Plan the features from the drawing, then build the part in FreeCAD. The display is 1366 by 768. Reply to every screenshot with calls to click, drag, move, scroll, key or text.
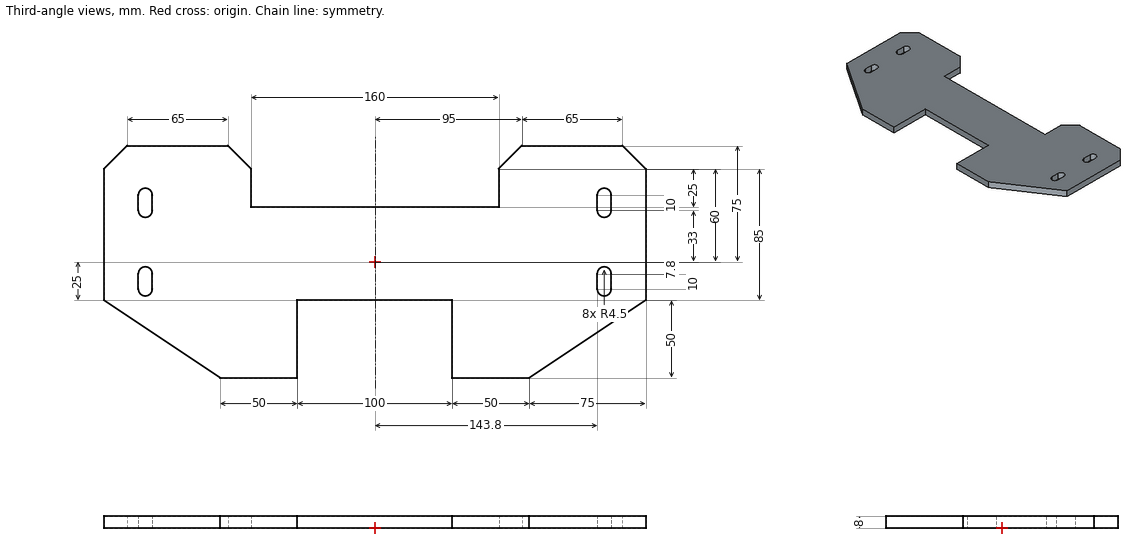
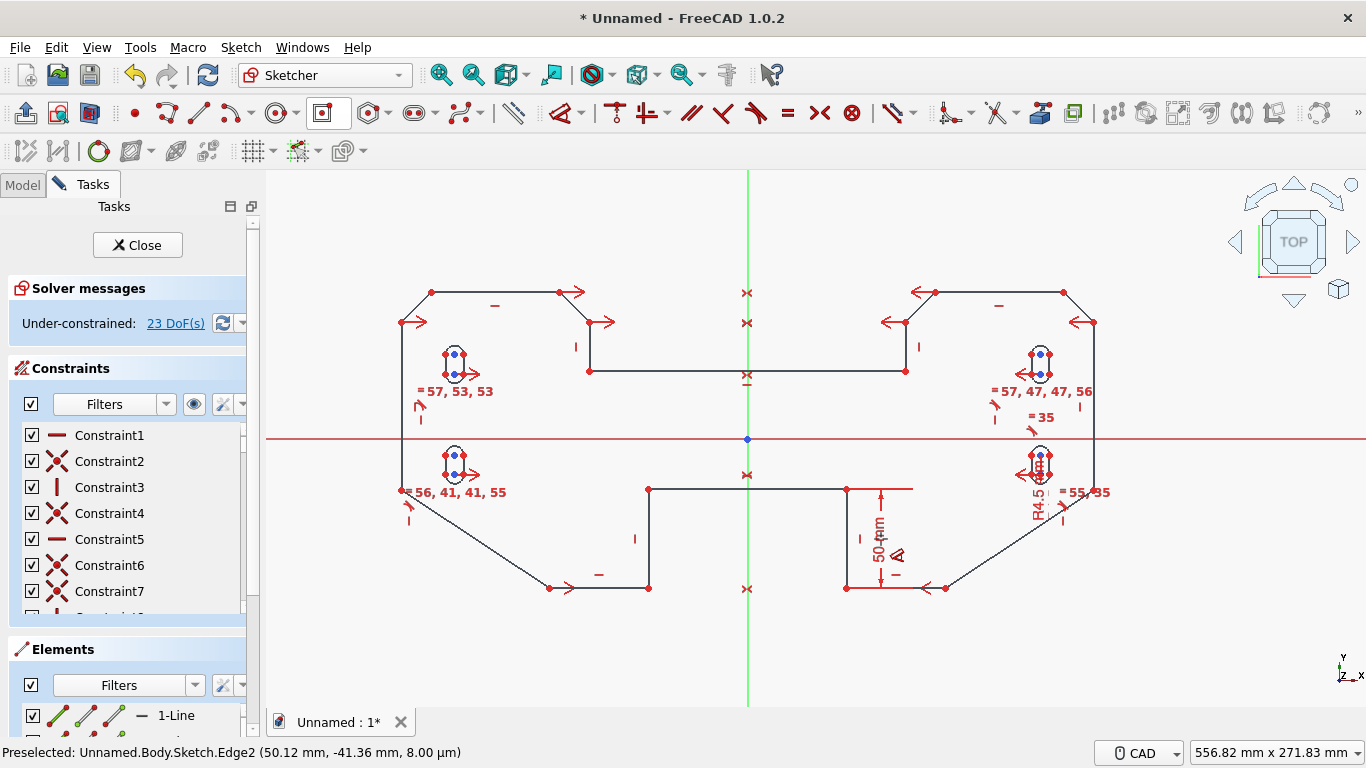
click(876, 588)
click(896, 622)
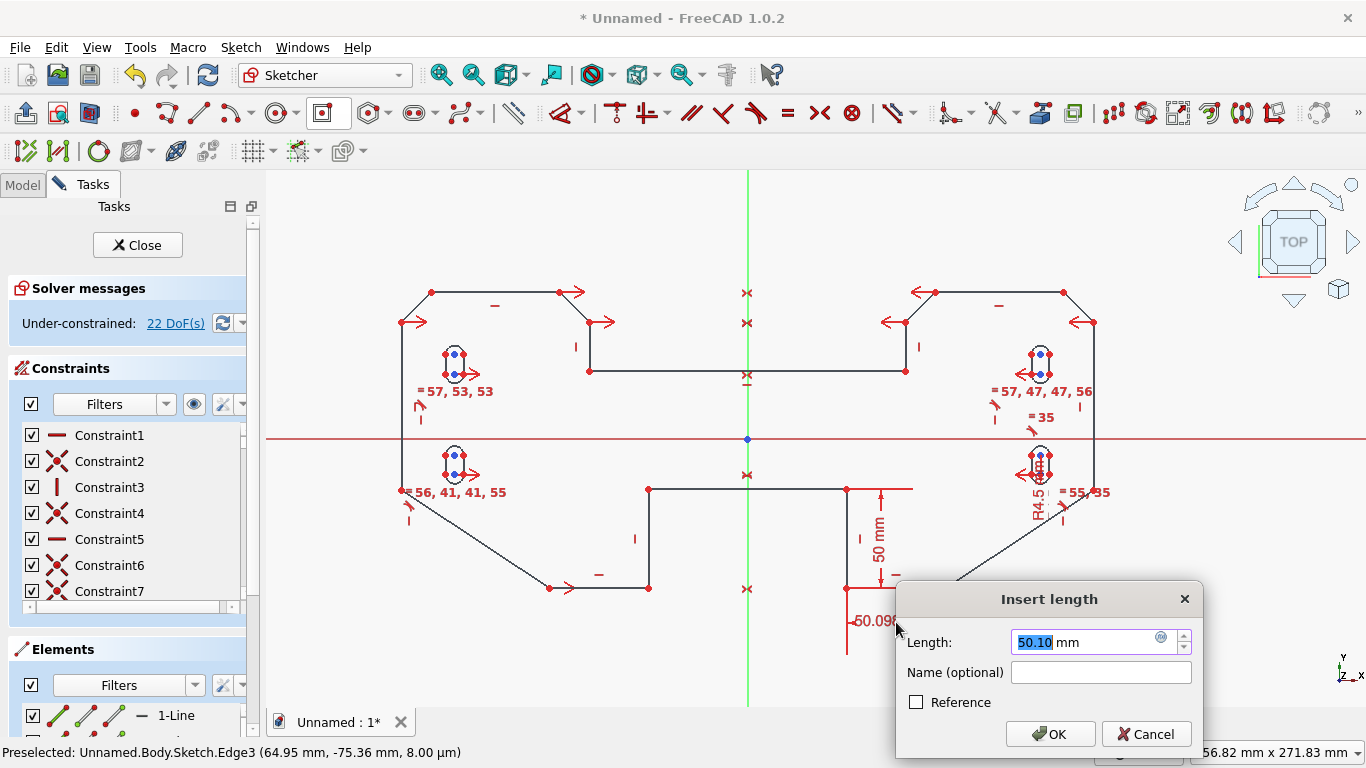
text(50)
key(Return)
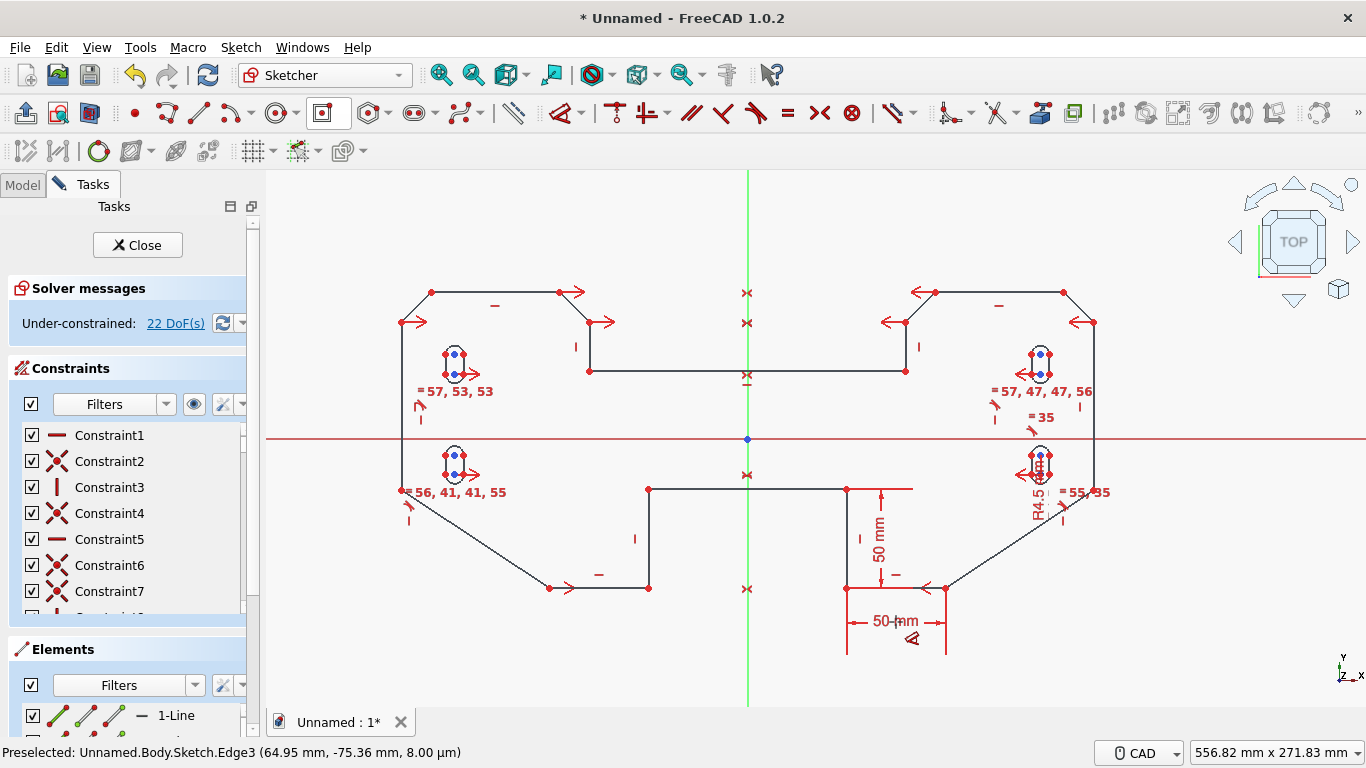
click(1094, 440)
click(1128, 406)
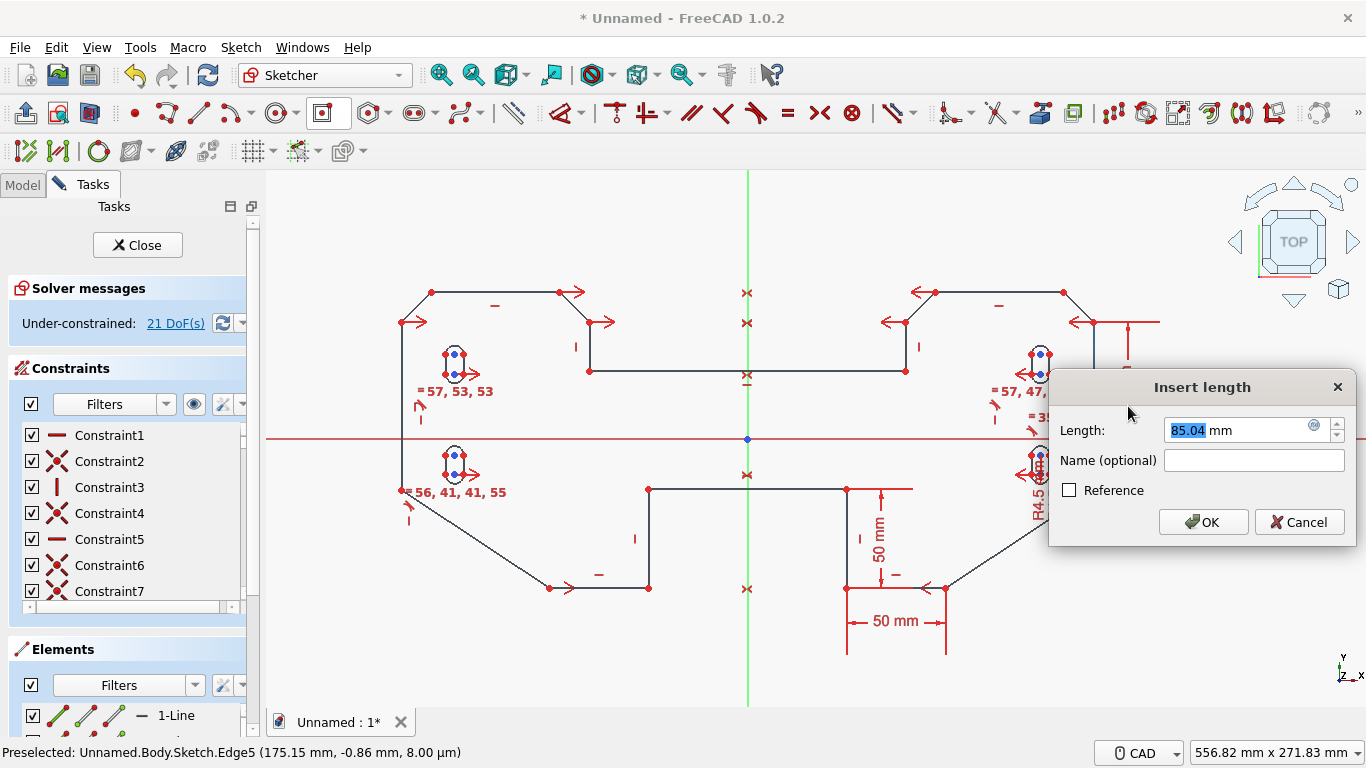
text(85)
key(Return)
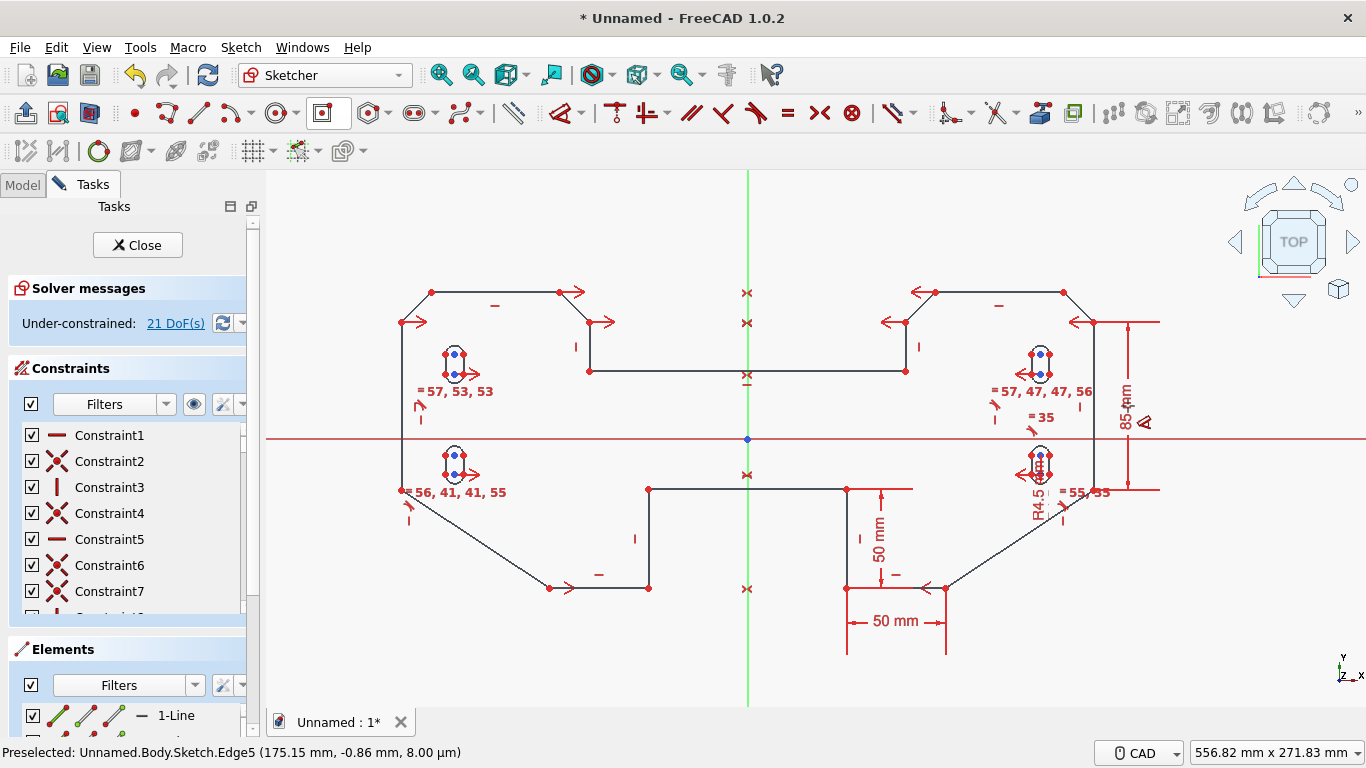
click(1025, 292)
click(1000, 258)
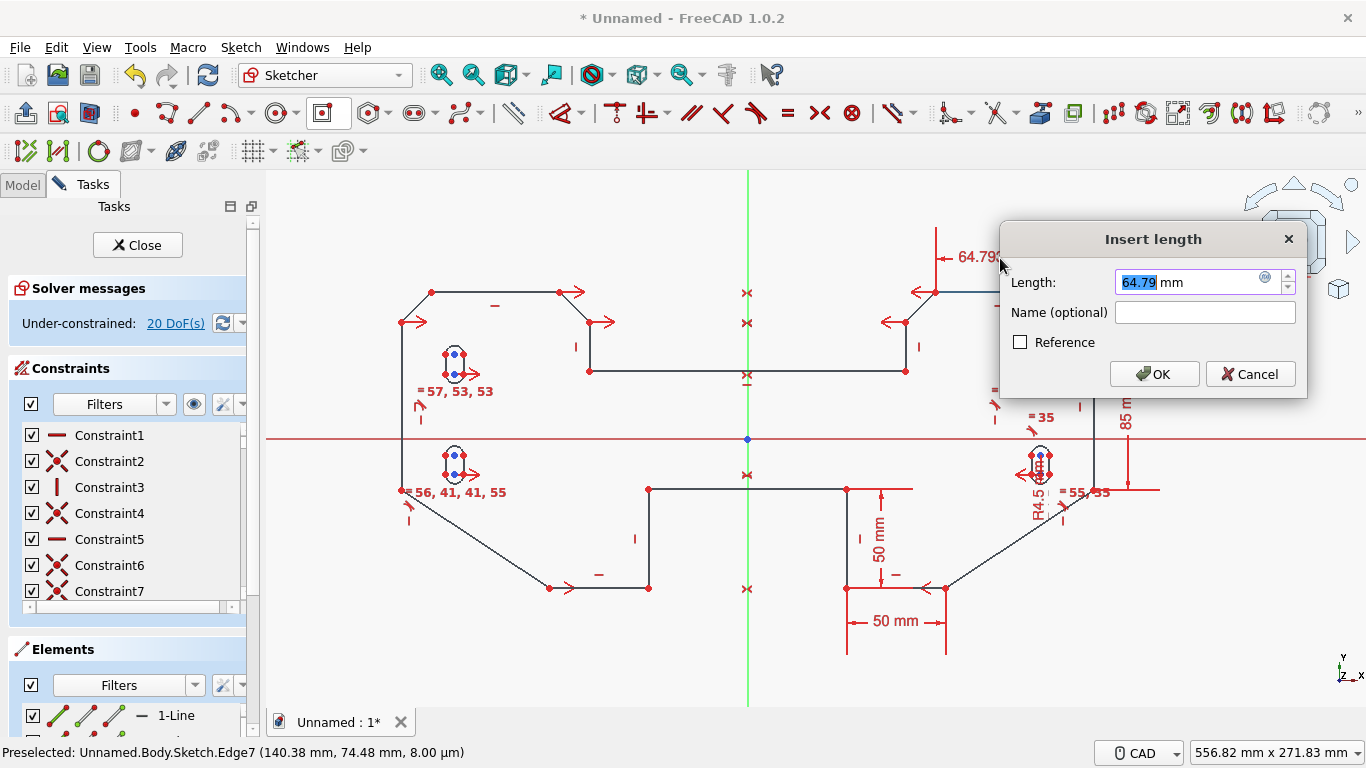
text(65)
key(Return)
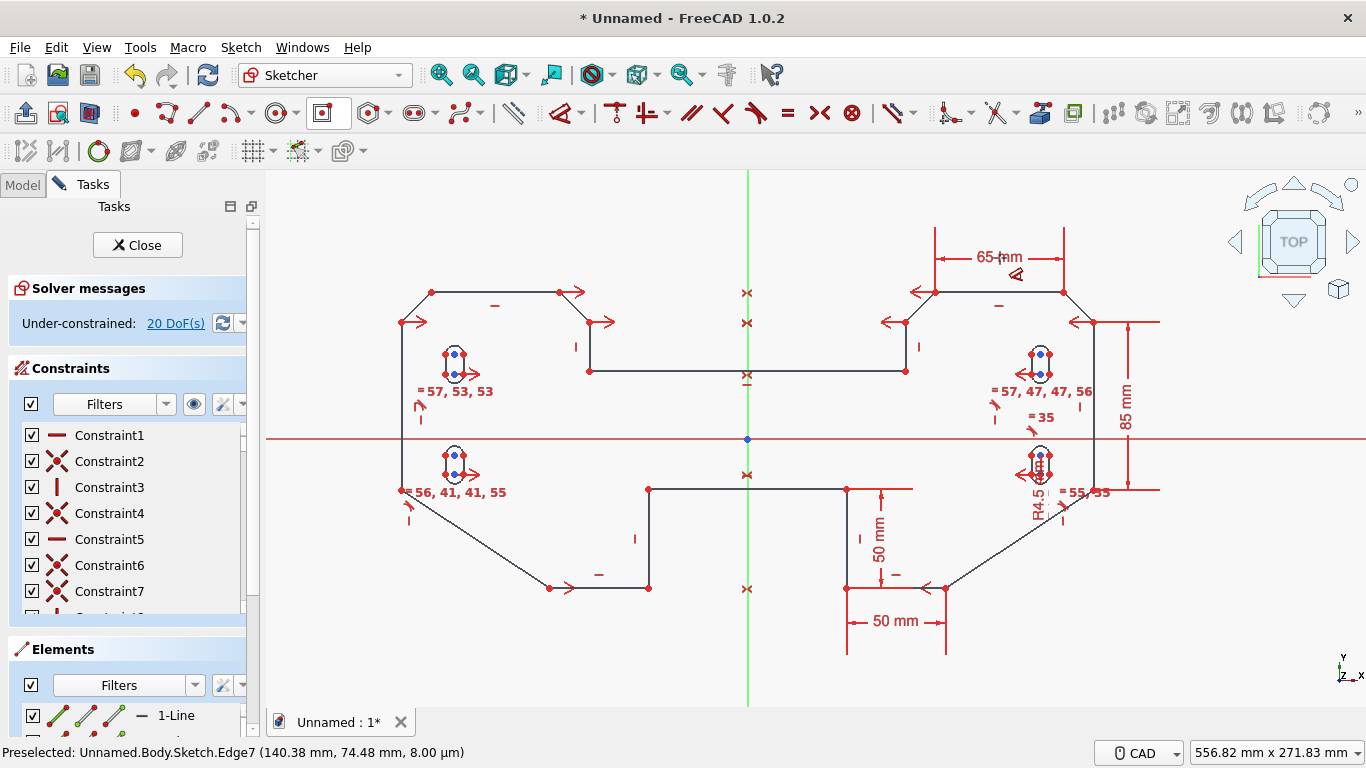
click(906, 337)
click(940, 347)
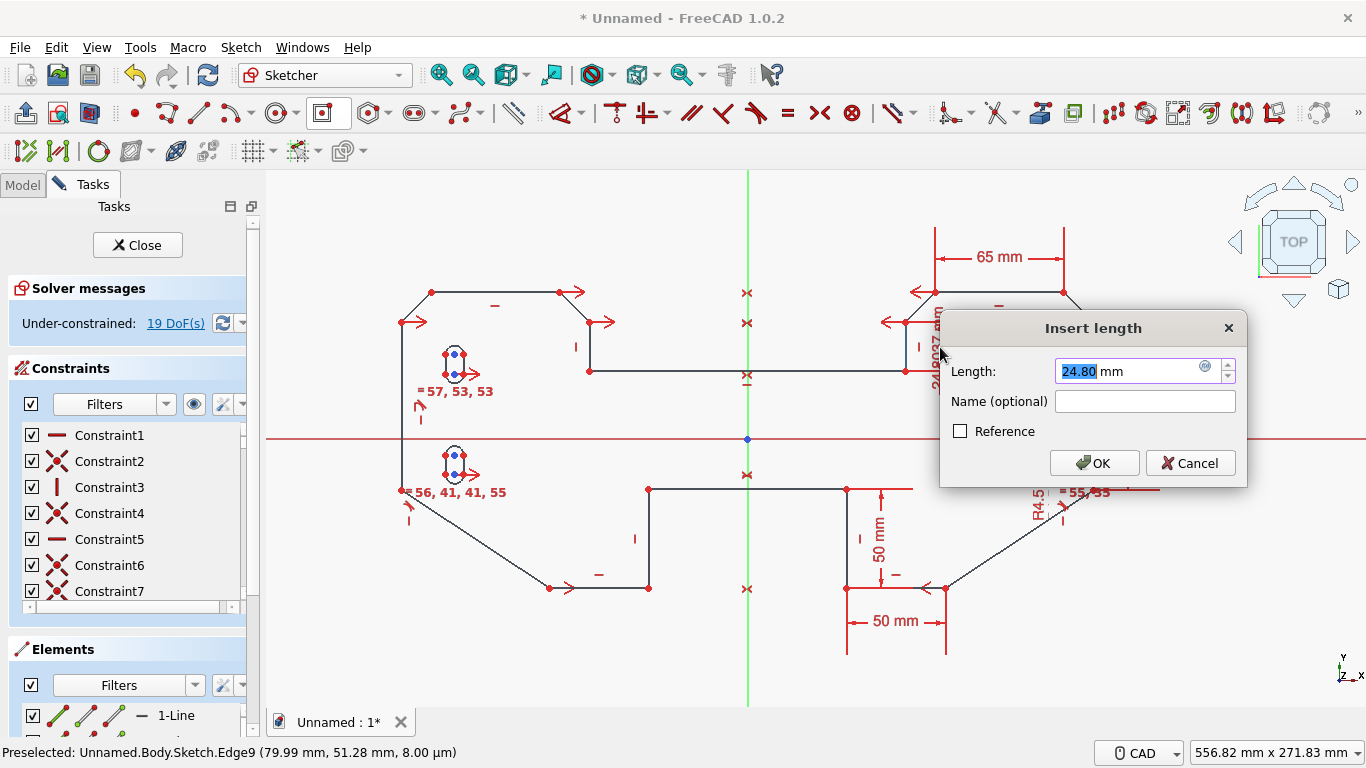
text(25)
key(Return)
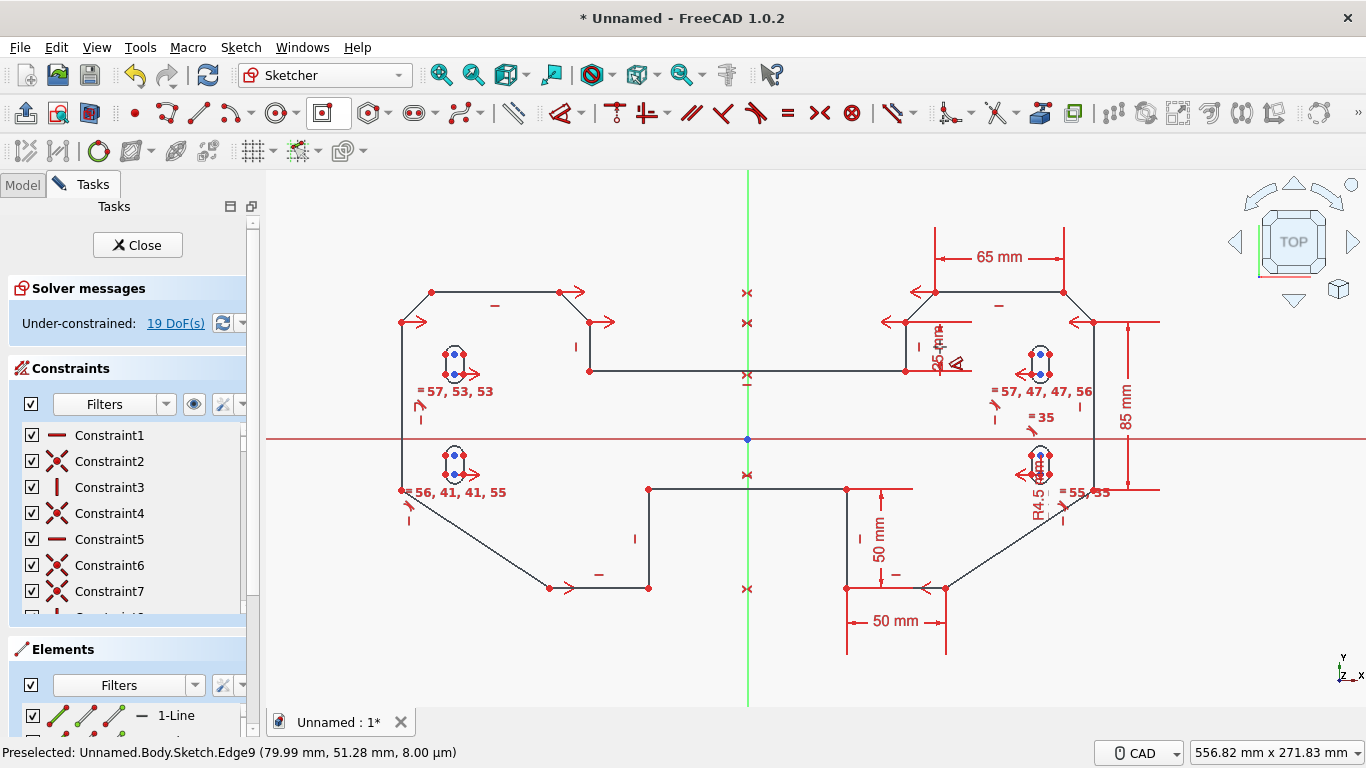
click(521, 292)
click(496, 258)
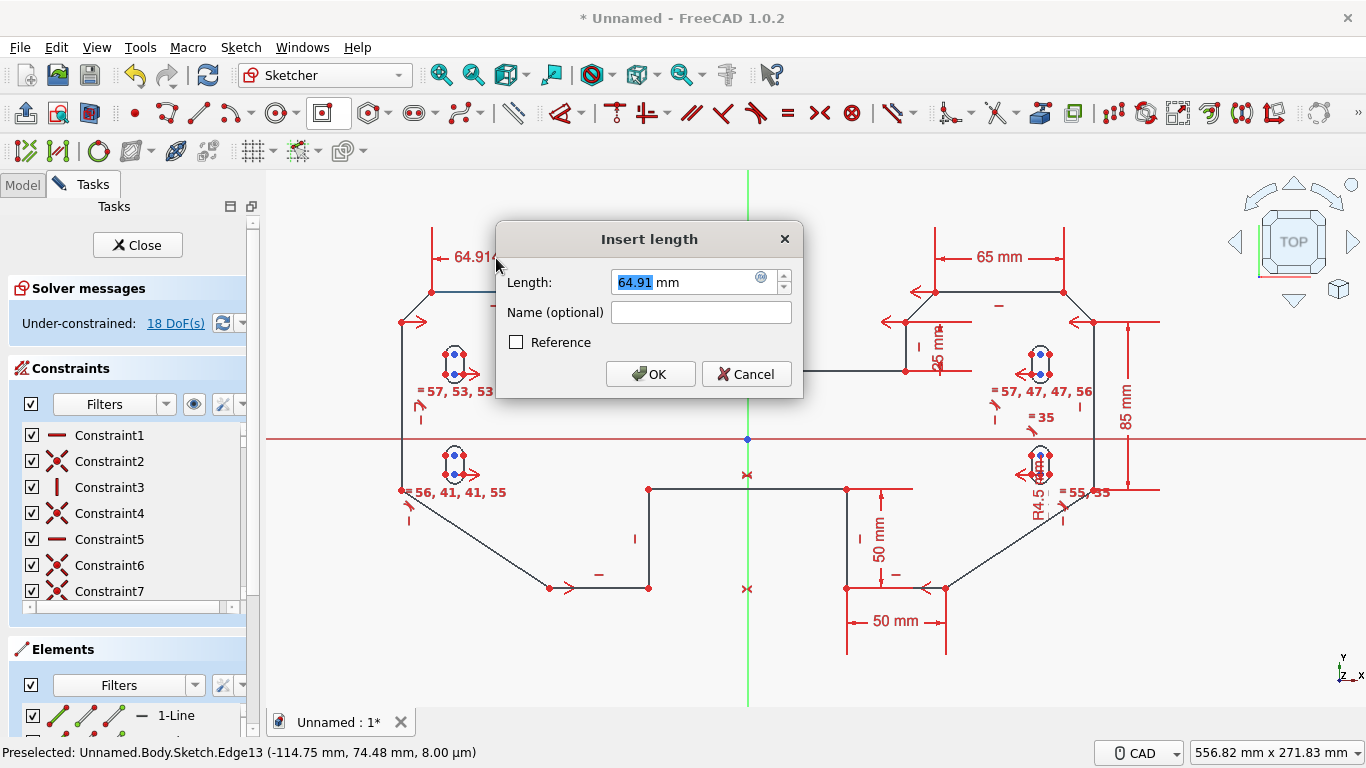
text(65)
key(Return)